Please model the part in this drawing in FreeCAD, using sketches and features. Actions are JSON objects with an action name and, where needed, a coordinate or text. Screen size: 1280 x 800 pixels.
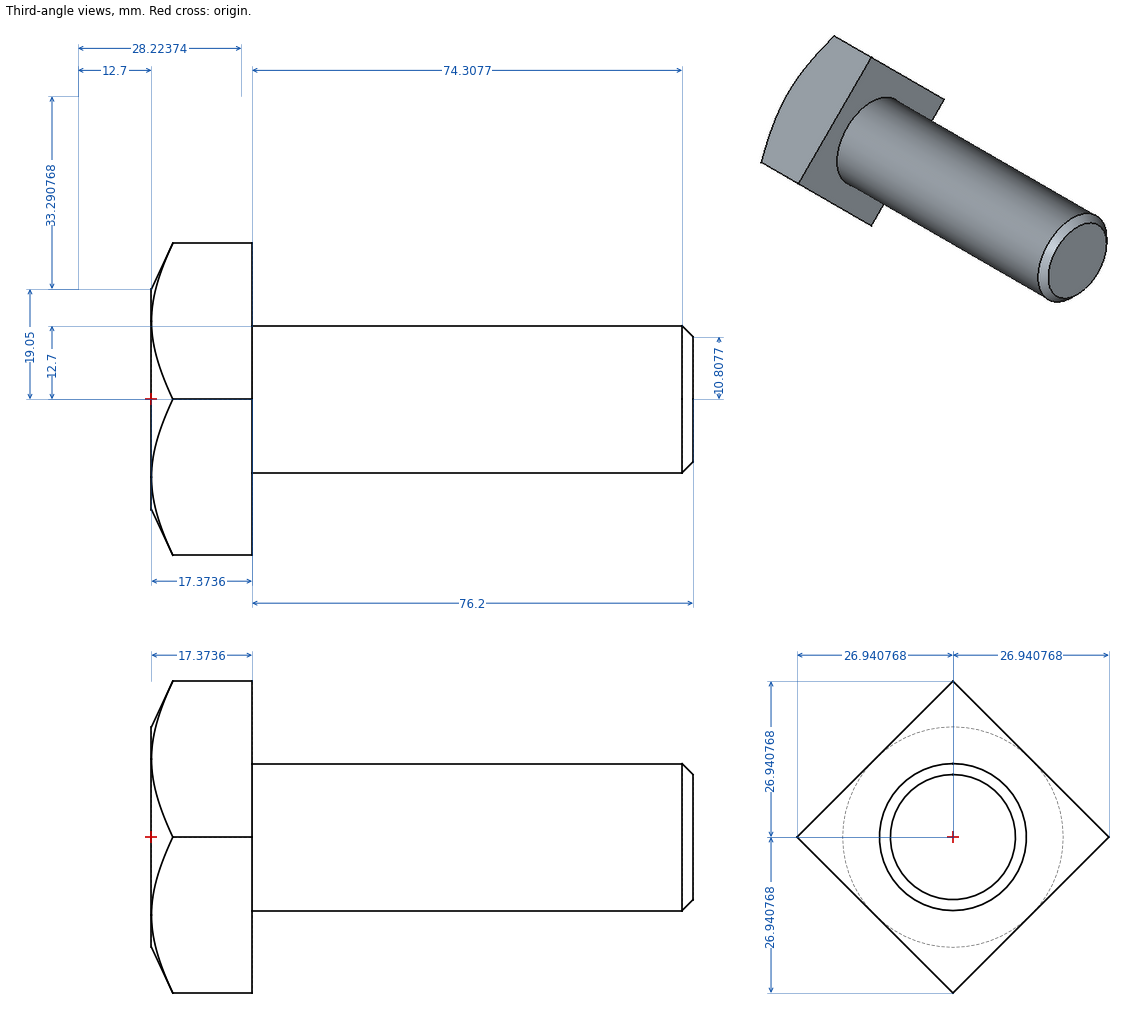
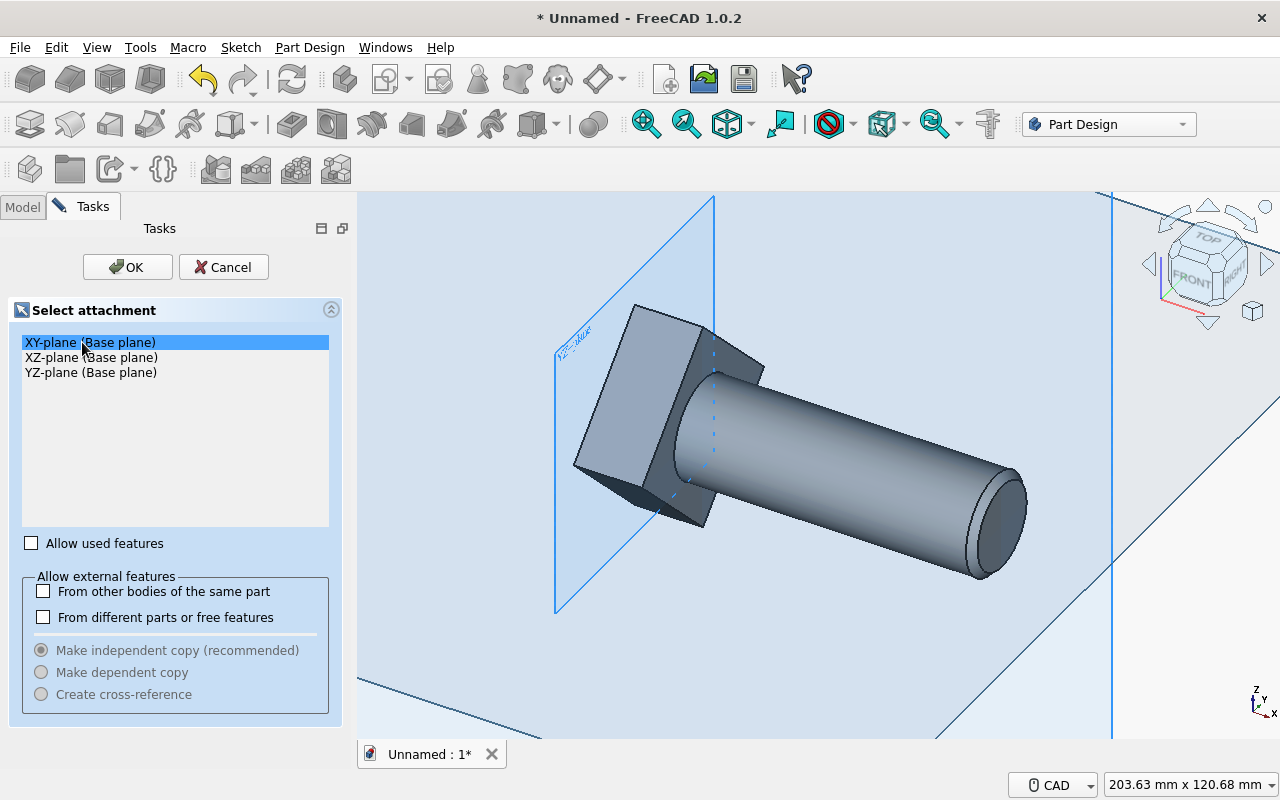
{"action": "left_click", "coordinate": [128, 267]}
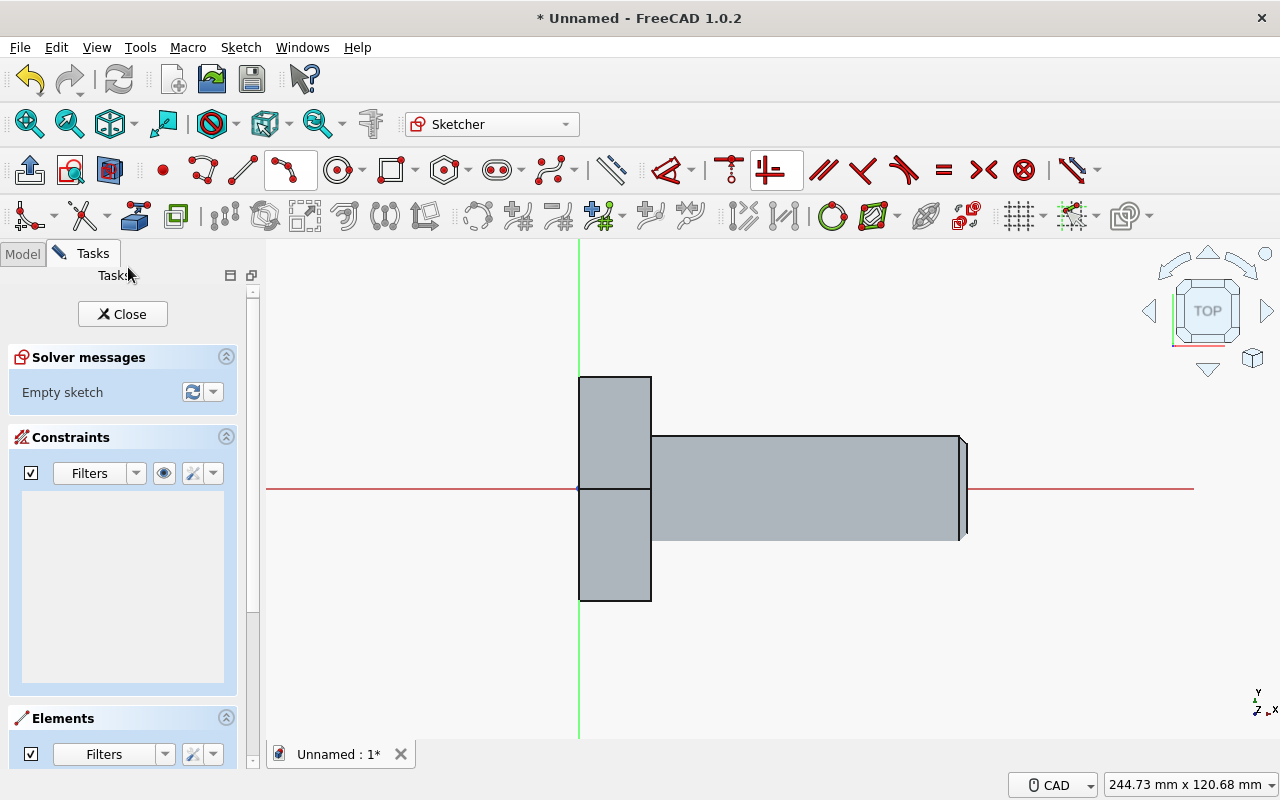
{"action": "left_click", "coordinate": [110, 170]}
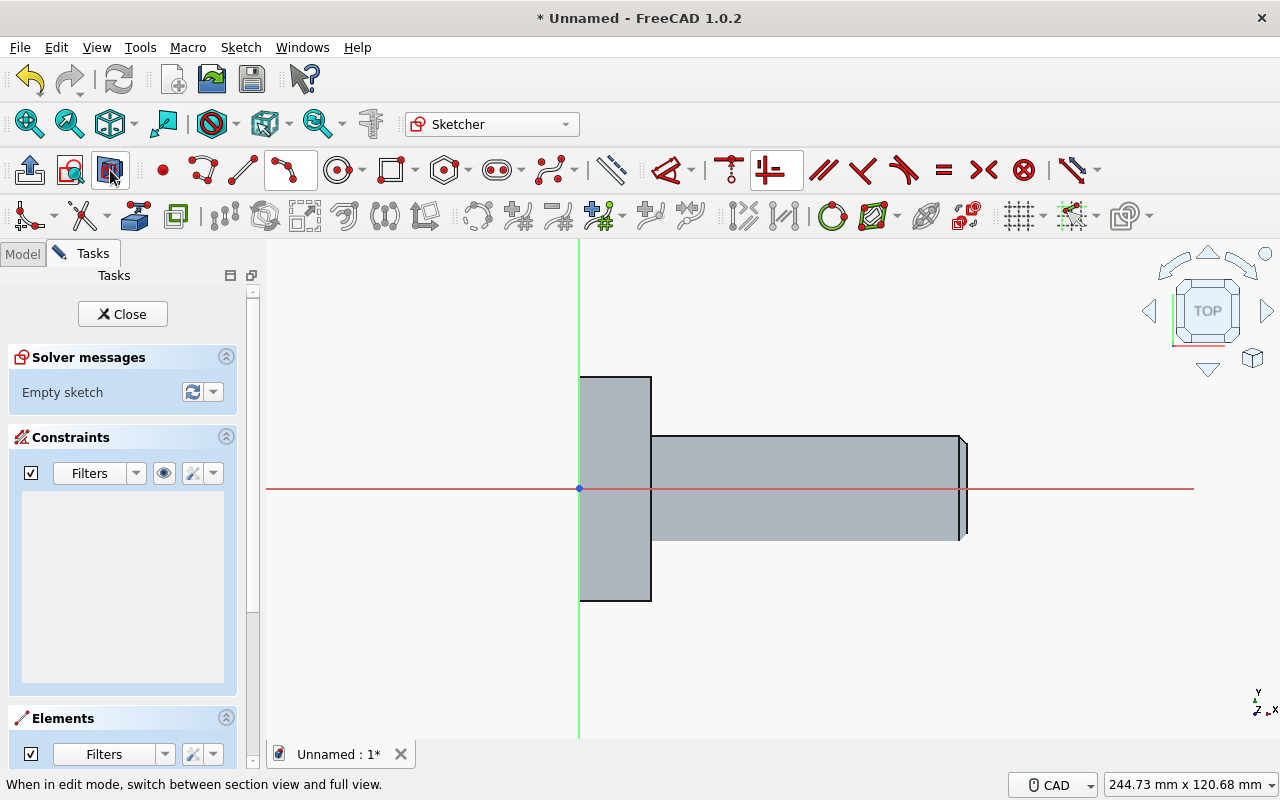
{"action": "scroll", "coordinate": [1115, 711], "scroll_direction": "down", "scroll_amount": 1}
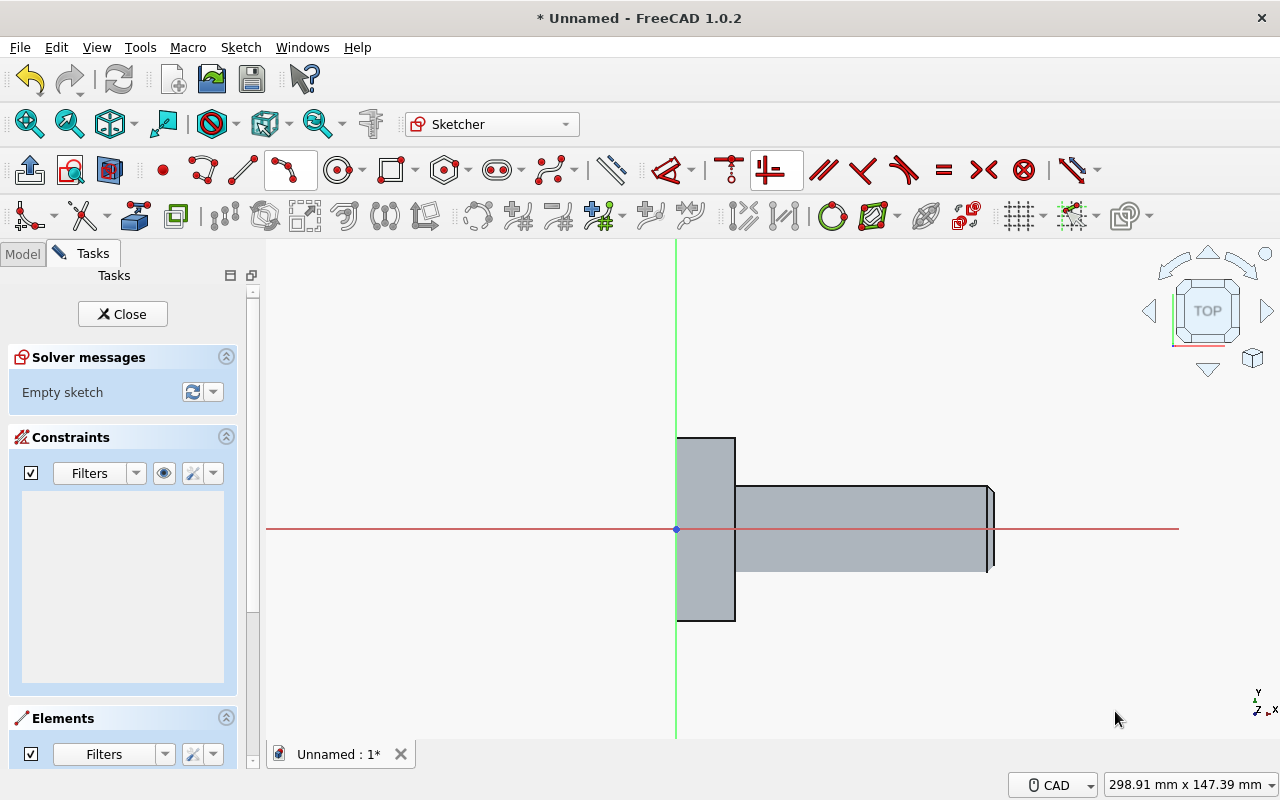
{"action": "scroll", "coordinate": [653, 382], "scroll_direction": "up", "scroll_amount": 3}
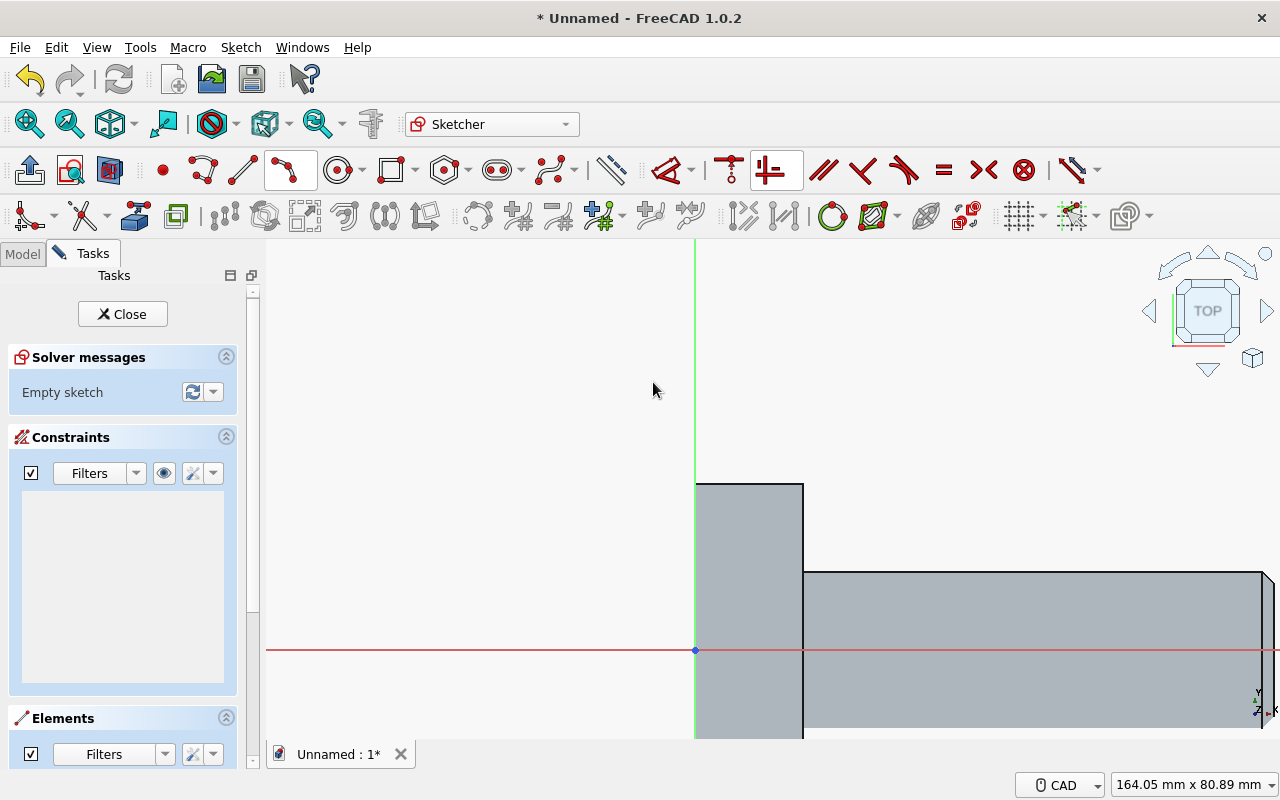
{"action": "left_click", "coordinate": [204, 170]}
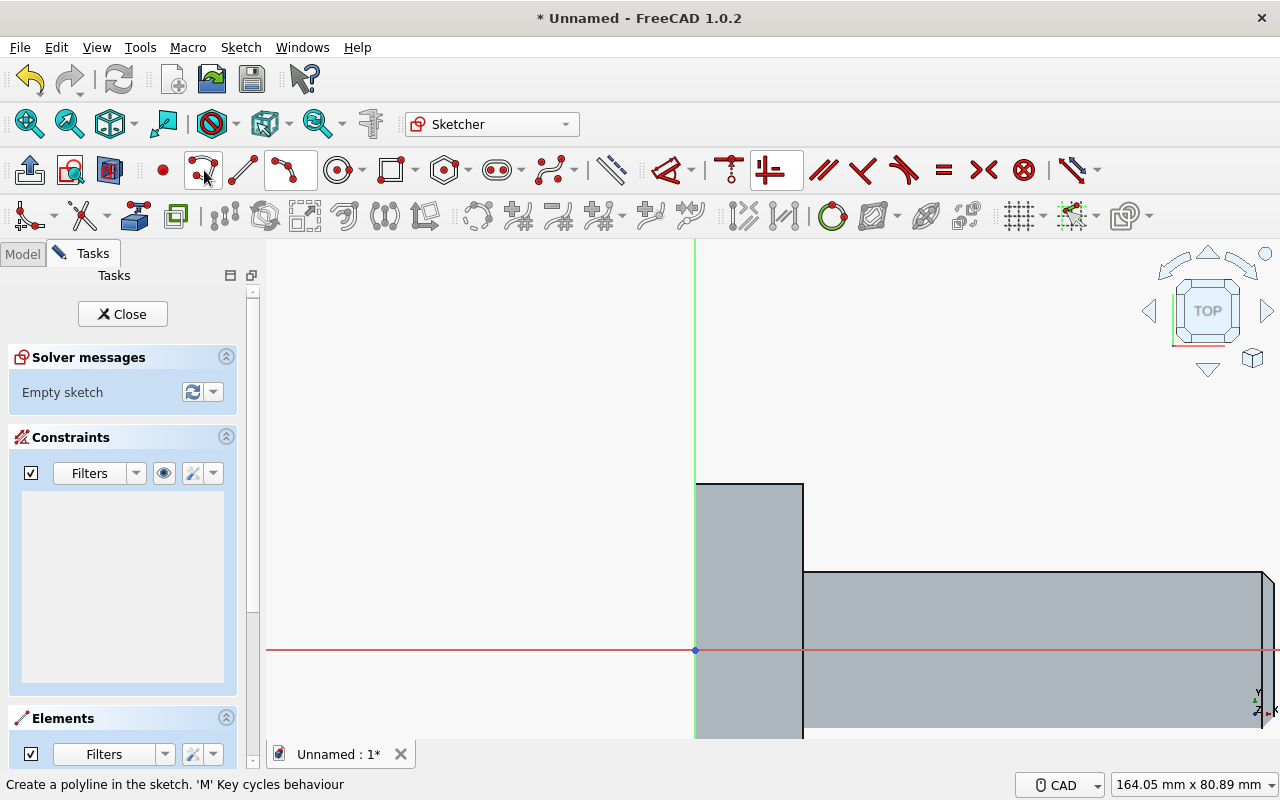
{"action": "left_click", "coordinate": [695, 533]}
{"action": "left_click", "coordinate": [791, 327]}
{"action": "left_click", "coordinate": [617, 327]}
{"action": "left_click", "coordinate": [617, 533]}
{"action": "left_click", "coordinate": [695, 534]}
{"action": "key", "text": "Escape"}
{"action": "key", "text": "Escape"}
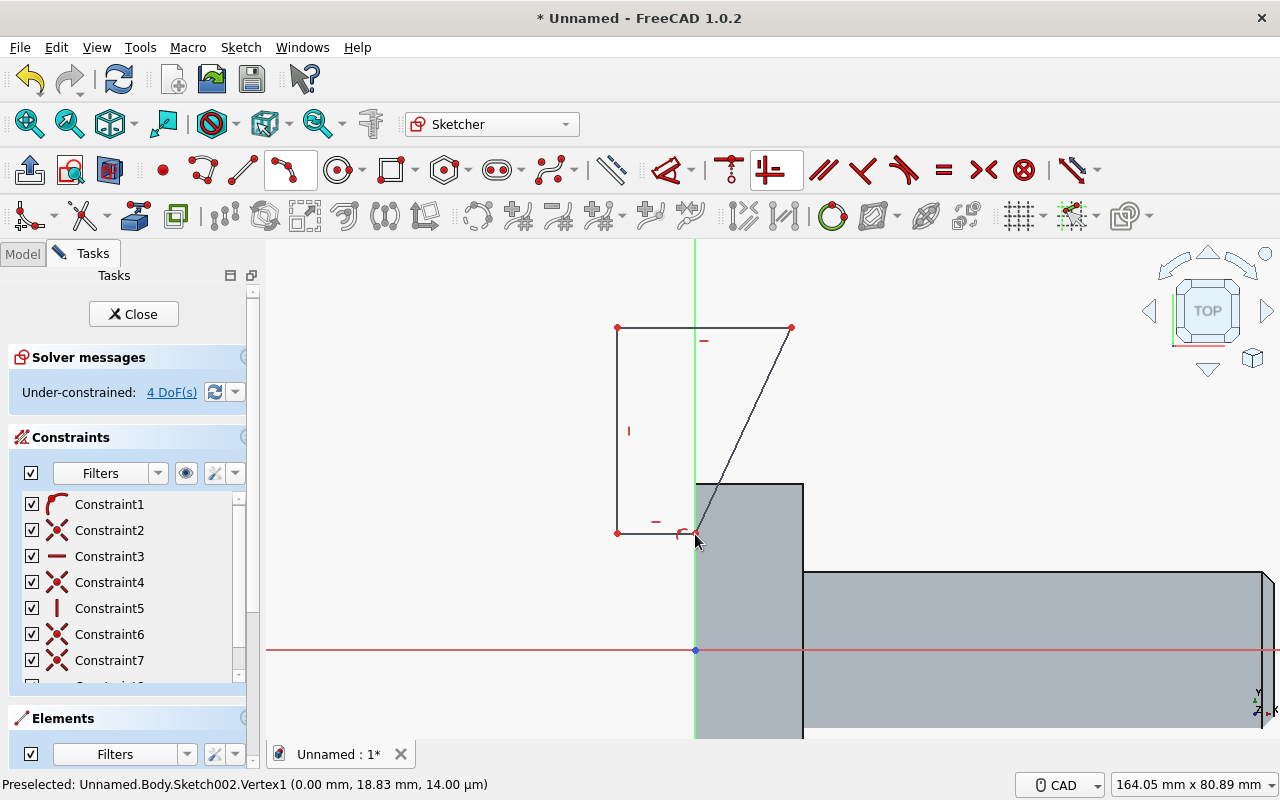
{"action": "left_click", "coordinate": [666, 170]}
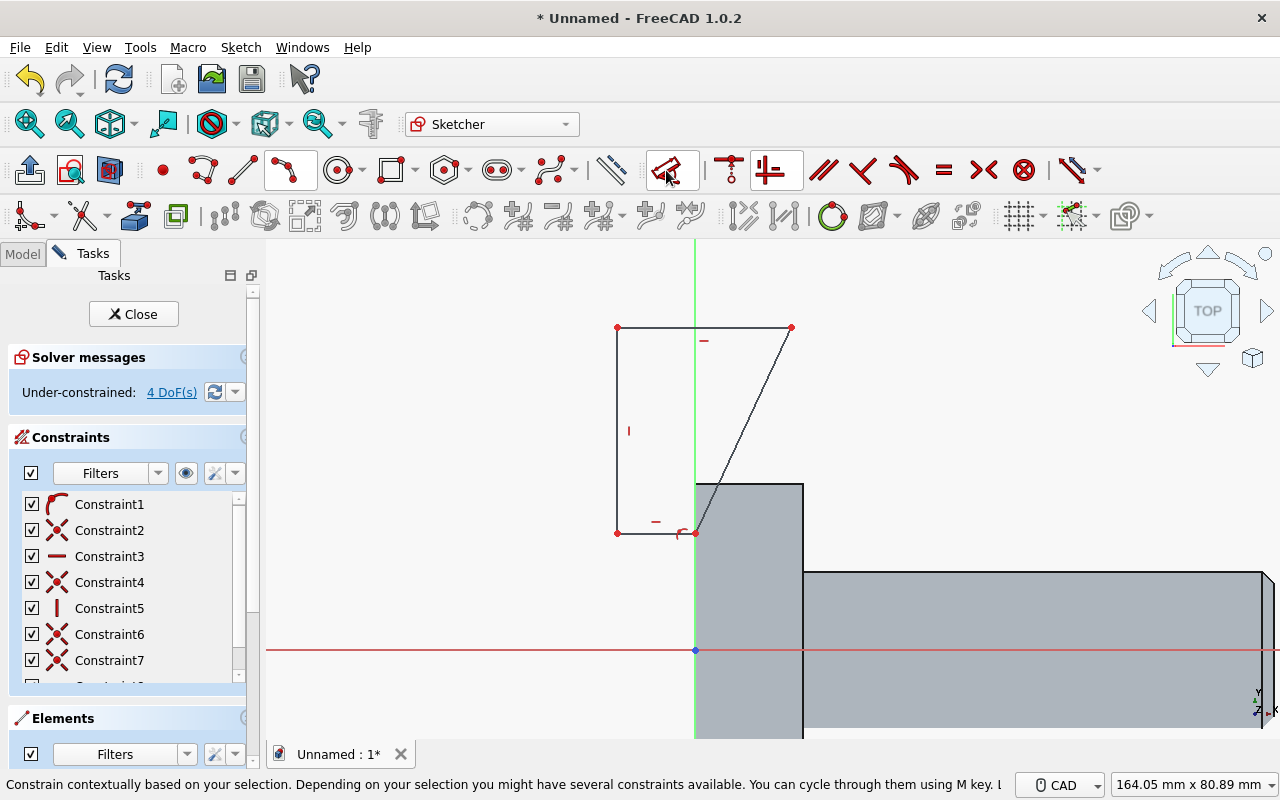
{"action": "left_click", "coordinate": [641, 534]}
{"action": "left_click", "coordinate": [656, 568]}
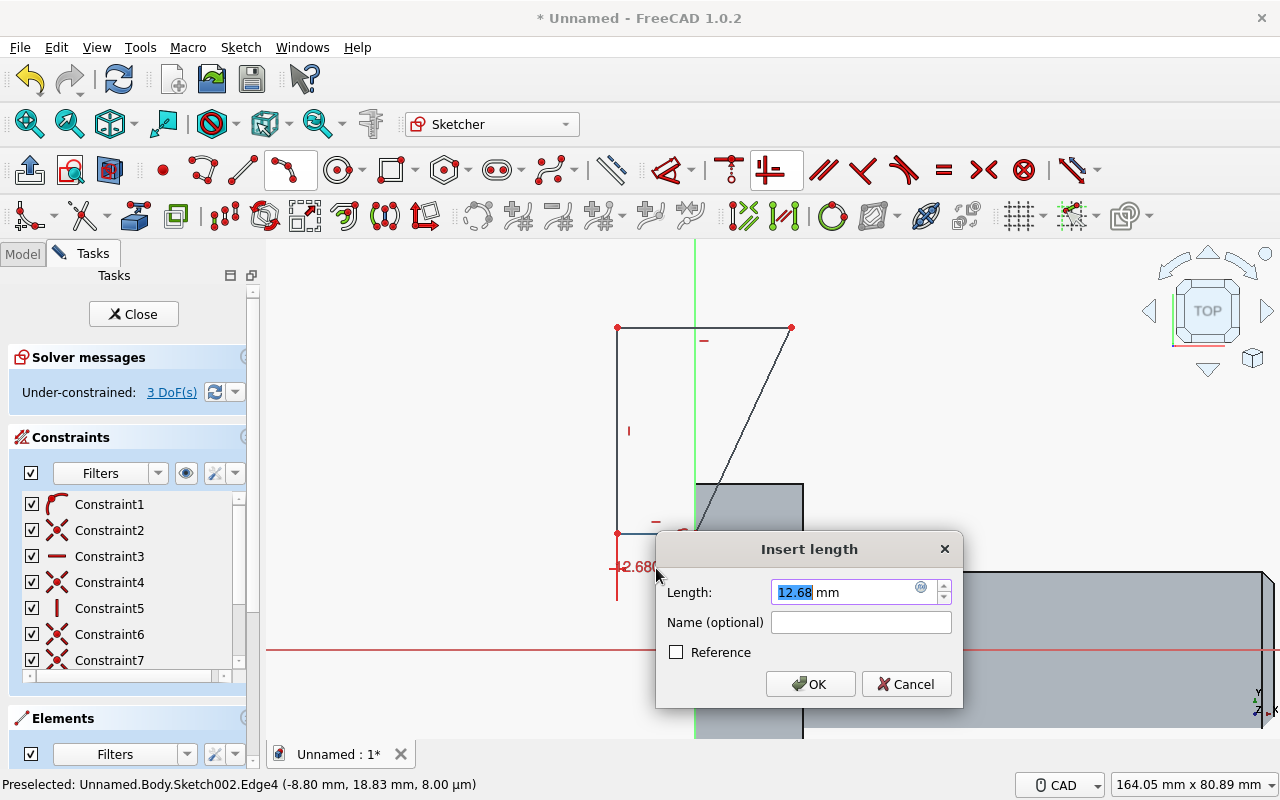
{"action": "type", "text": "12.7"}
{"action": "key", "text": "Return"}